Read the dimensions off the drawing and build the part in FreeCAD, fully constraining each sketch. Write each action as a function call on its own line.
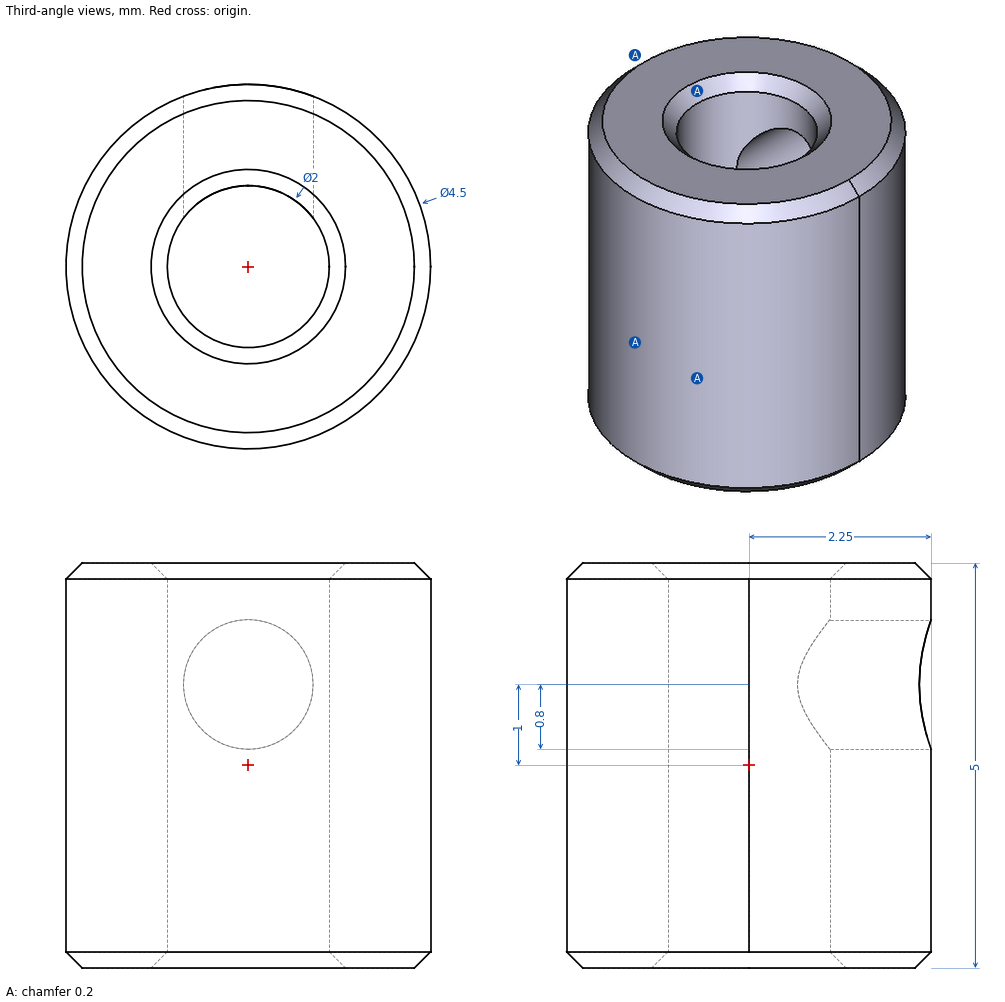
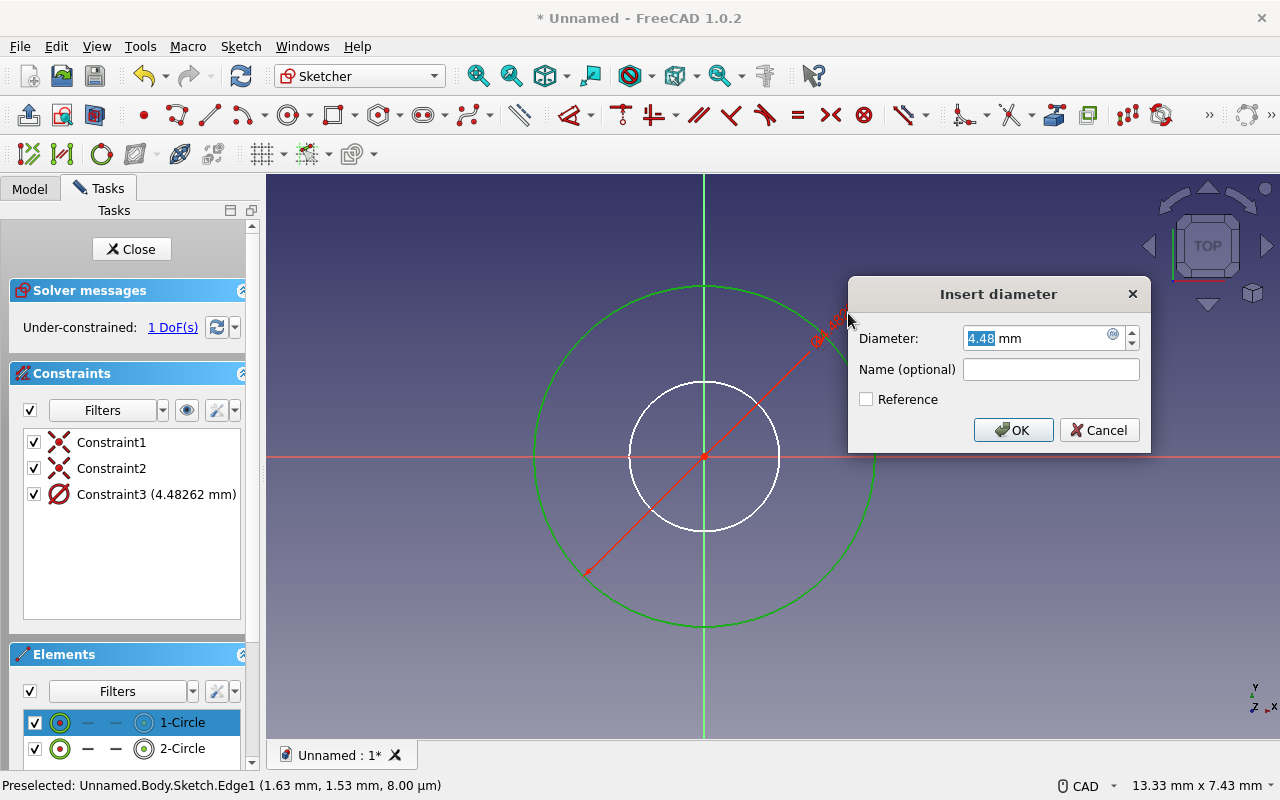
text(4.5)
key(Return)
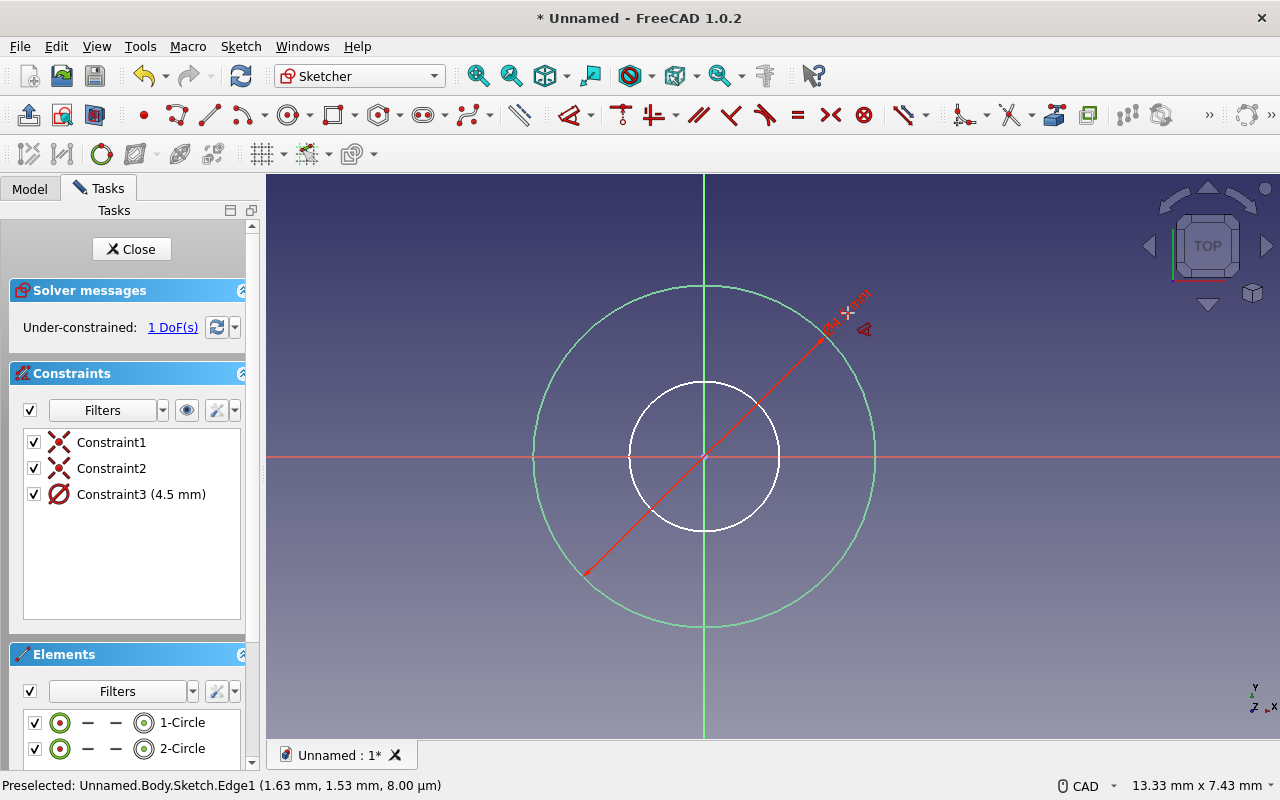
click(757, 403)
click(779, 380)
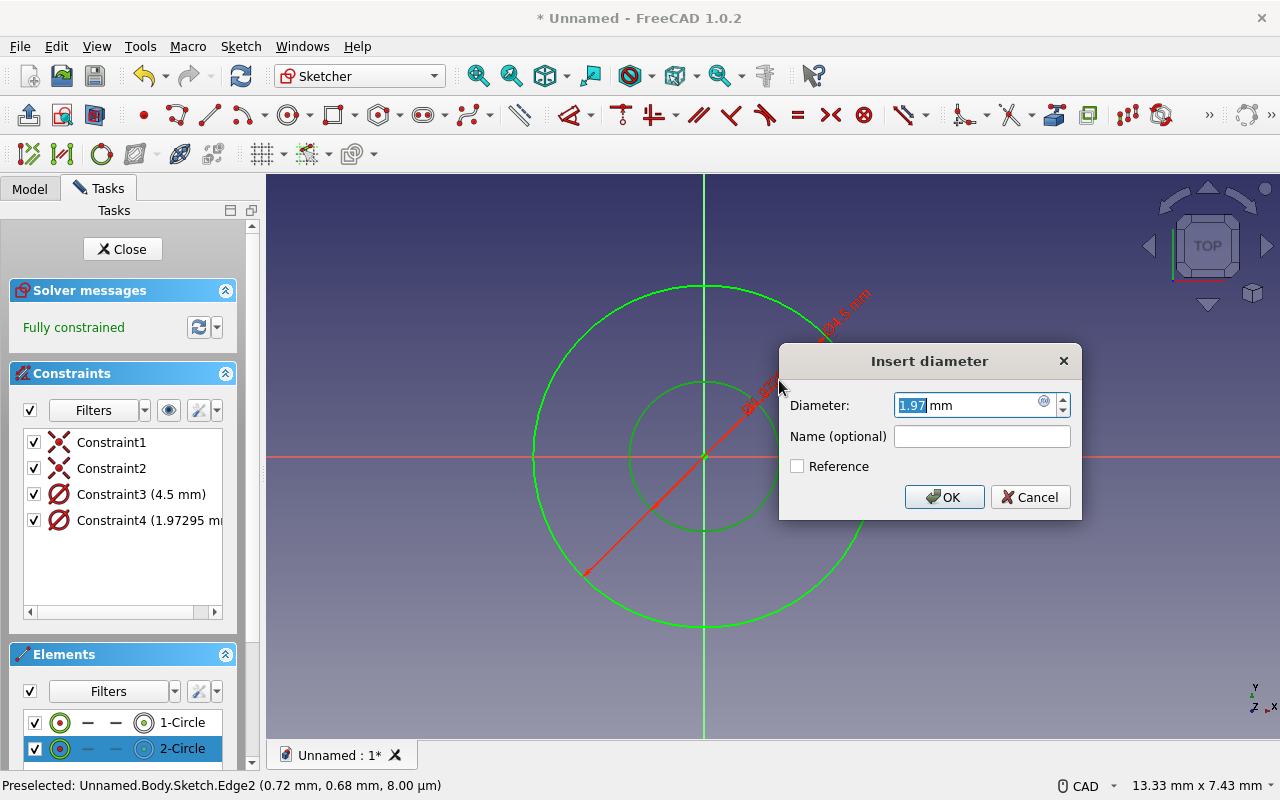
text(2)
key(Return)
key(Escape)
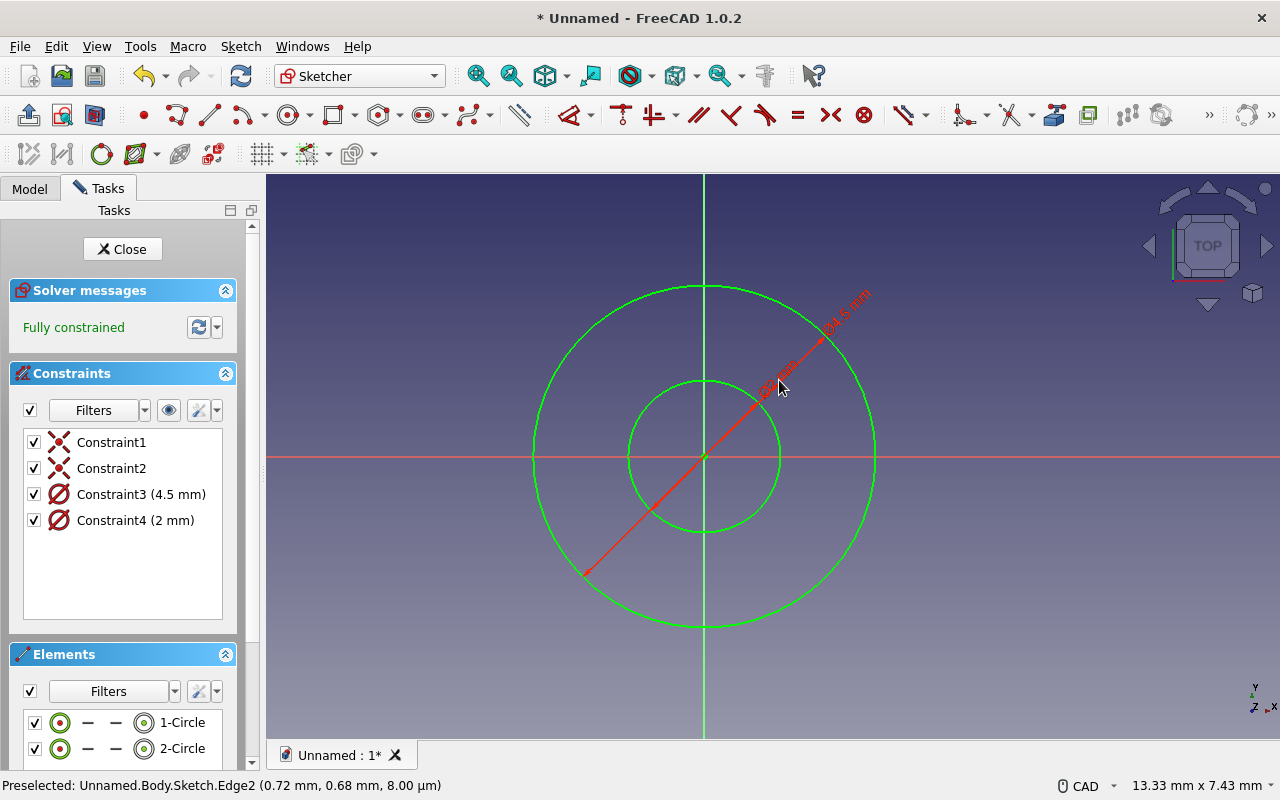
click(123, 249)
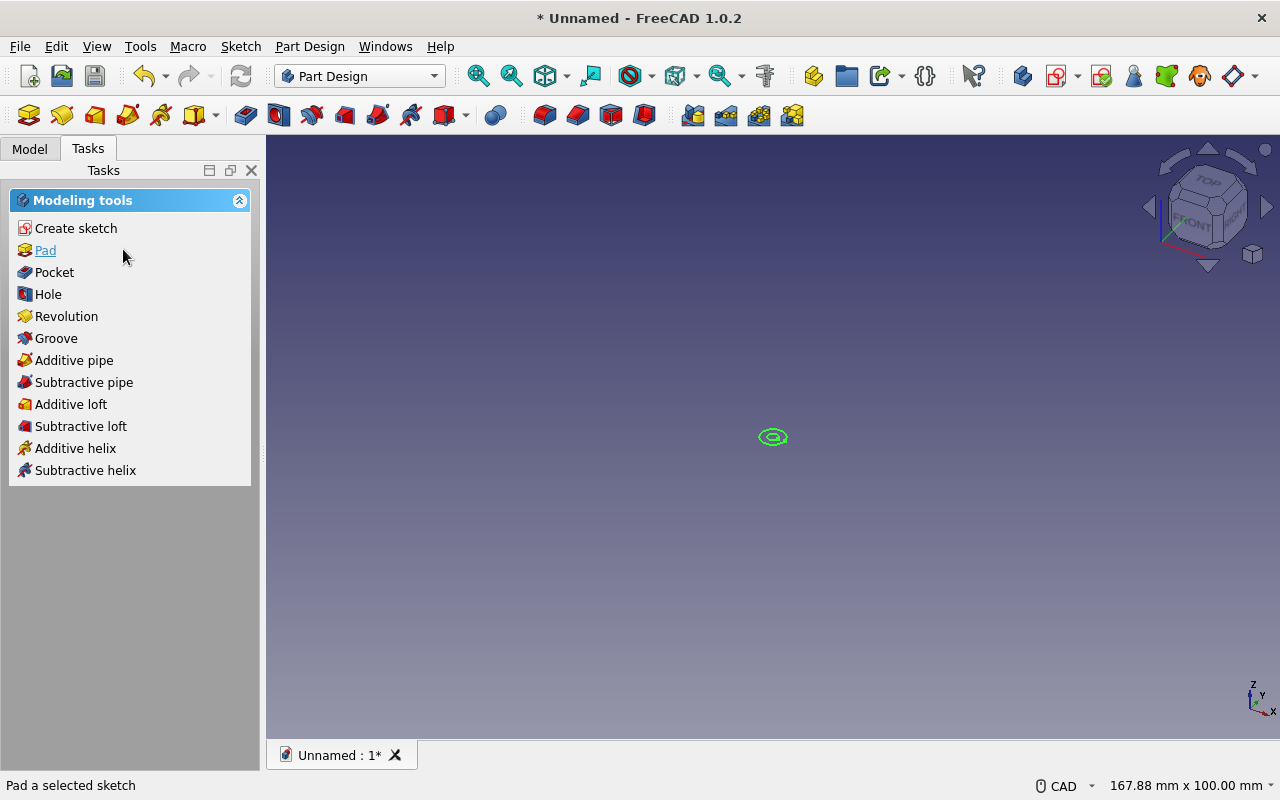
click(29, 116)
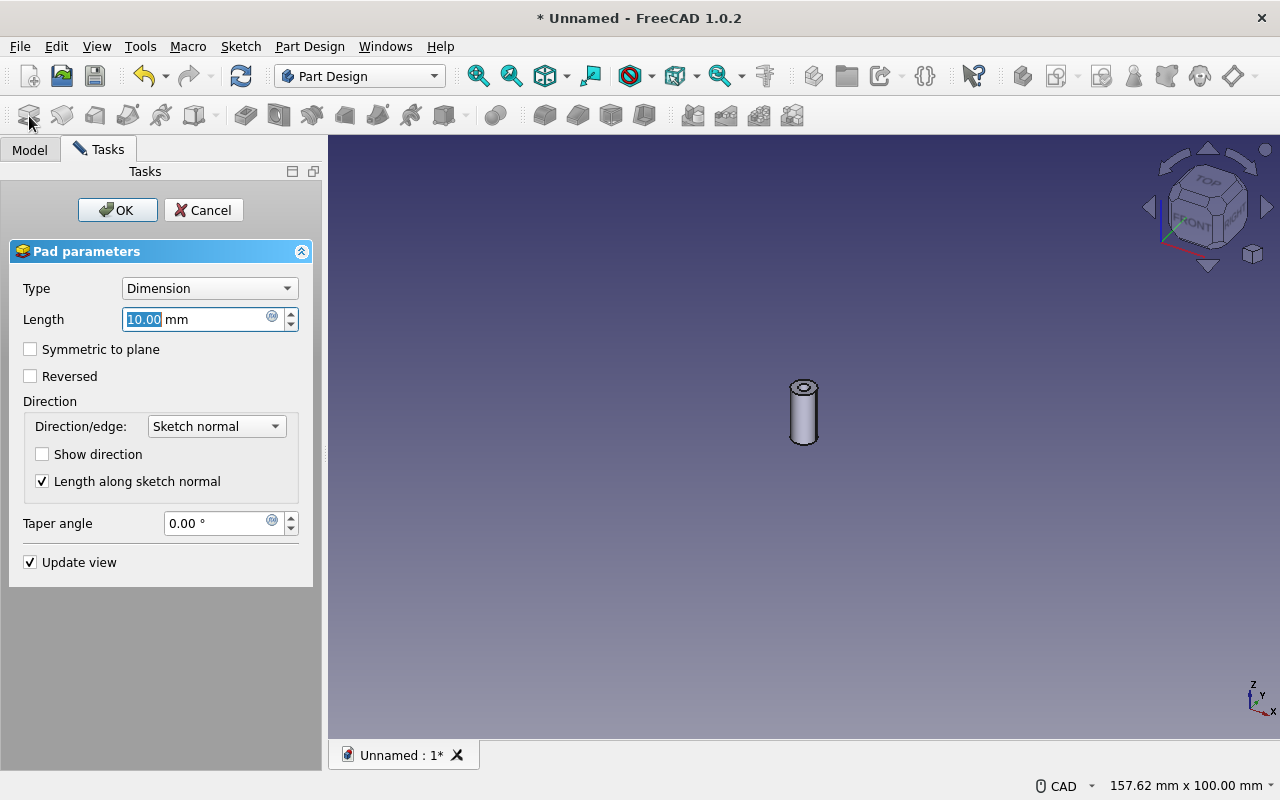
text(5)
key(Tab)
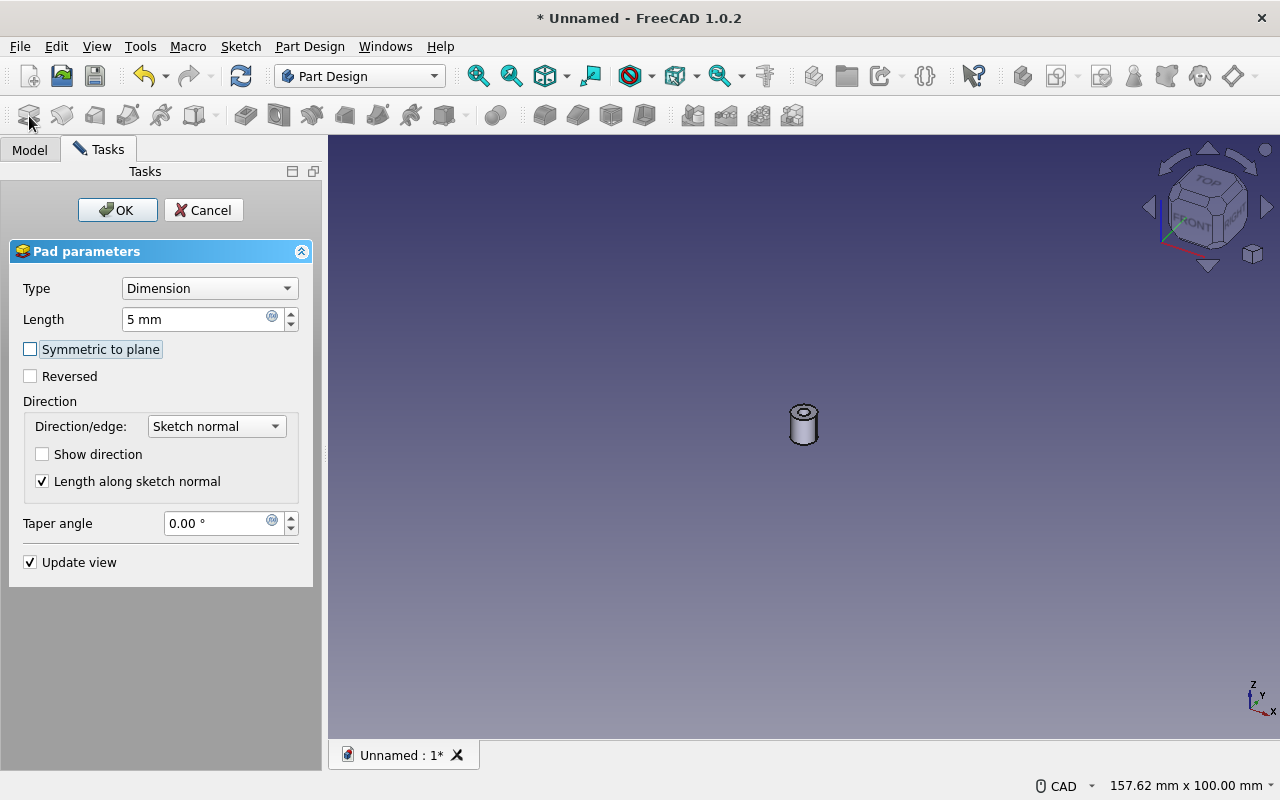
click(31, 349)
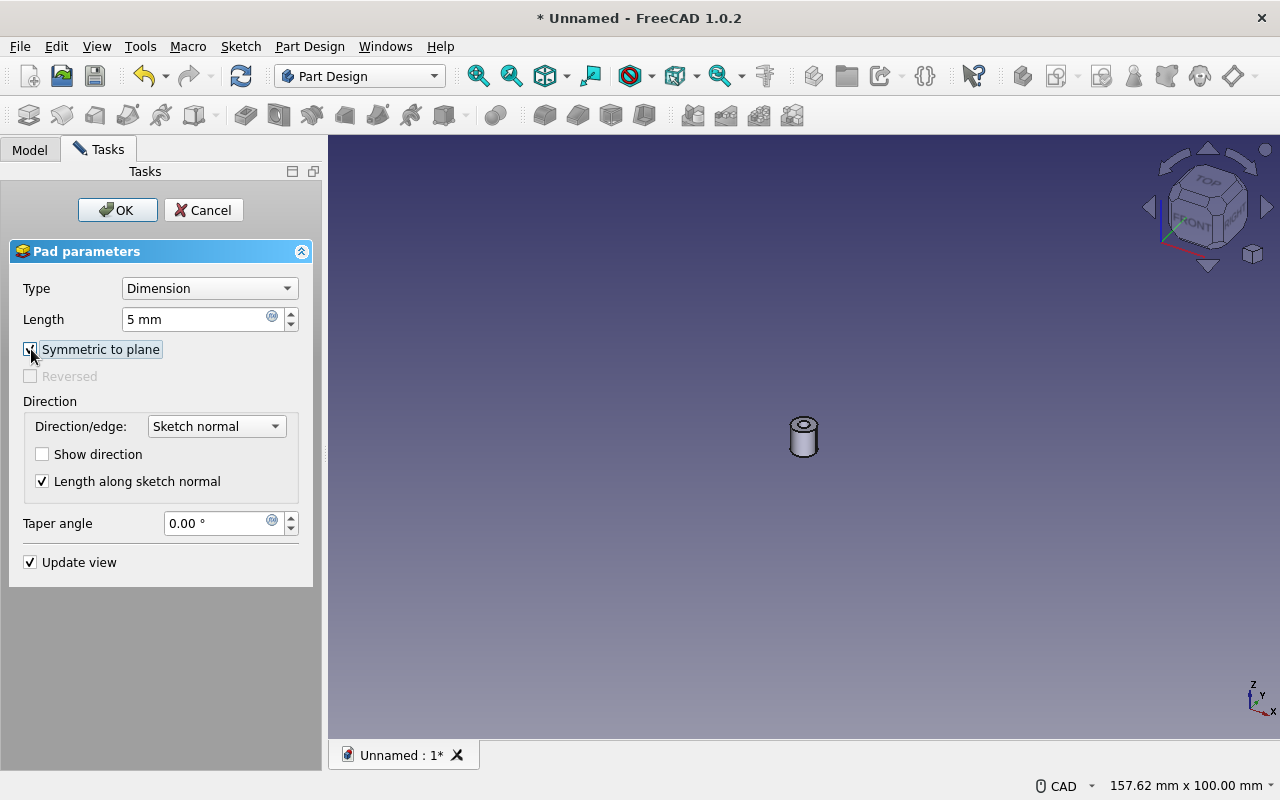
click(118, 210)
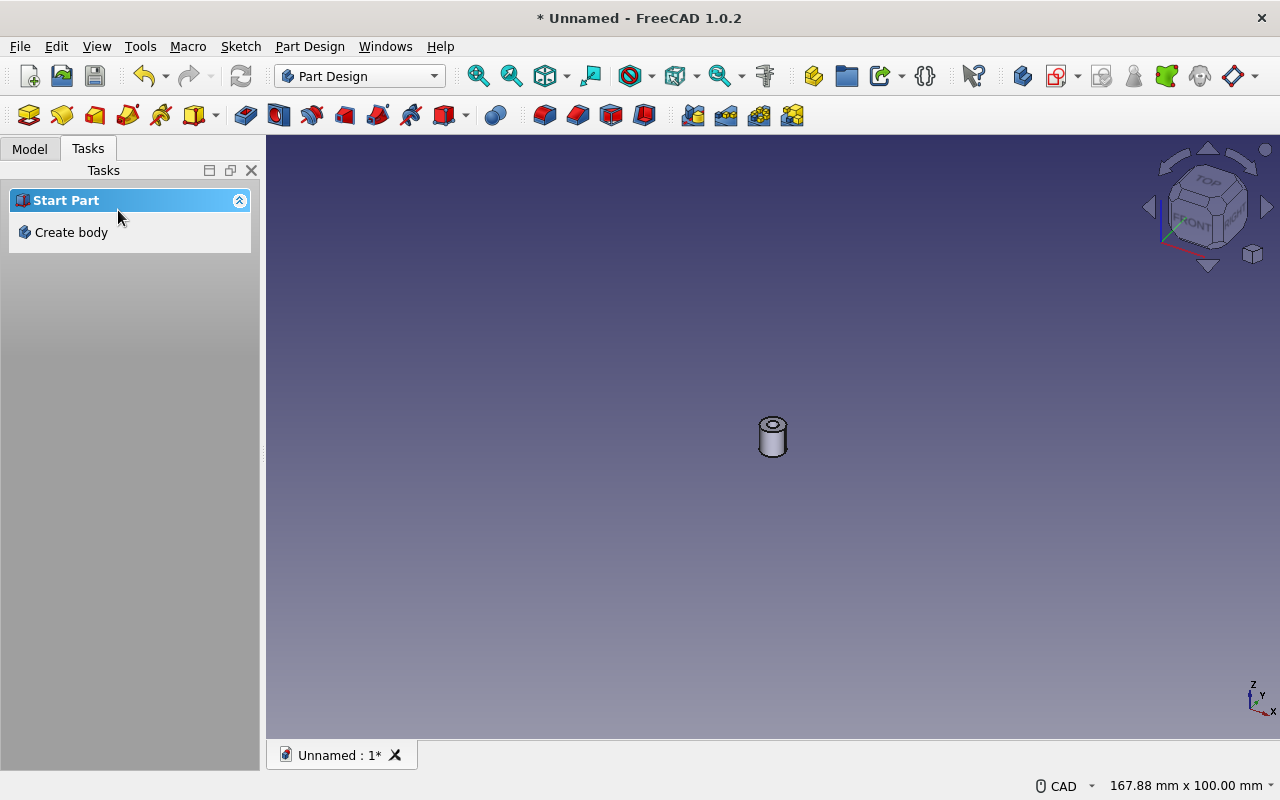
click(479, 76)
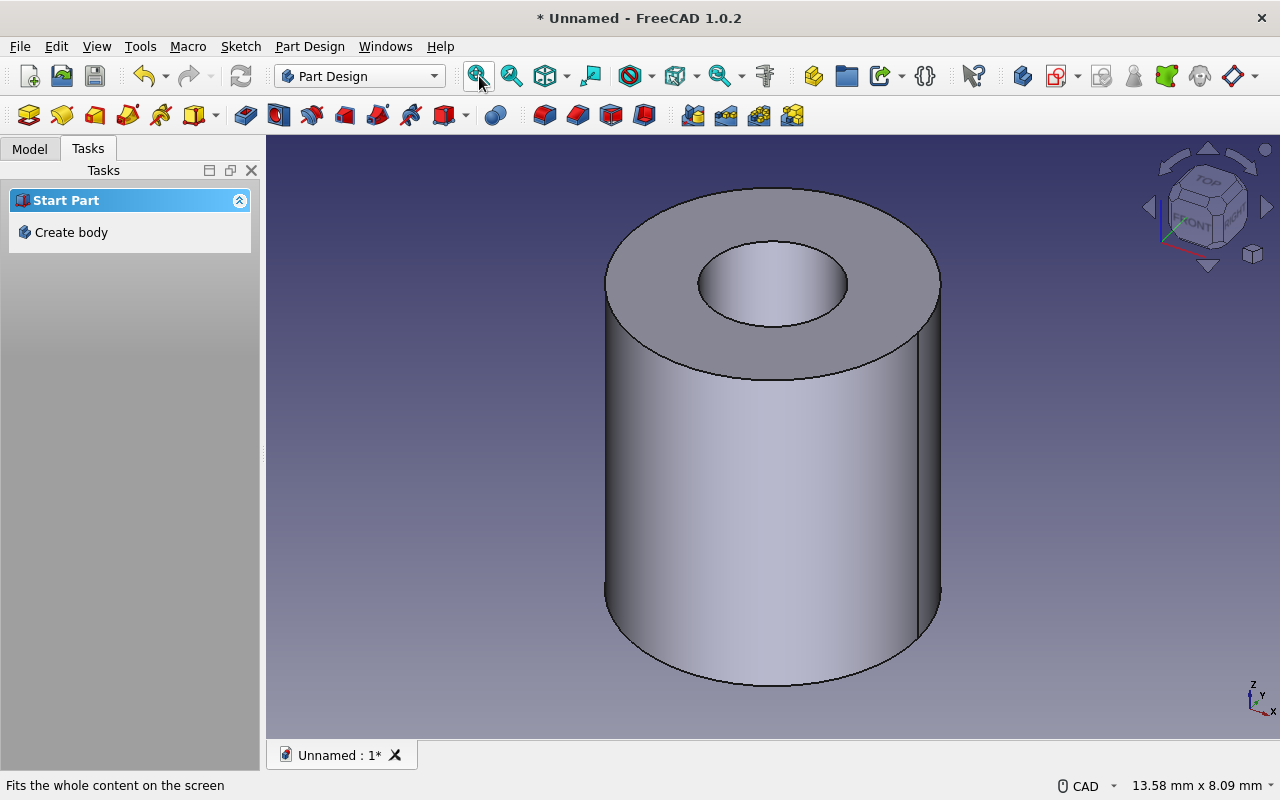
click(606, 293)